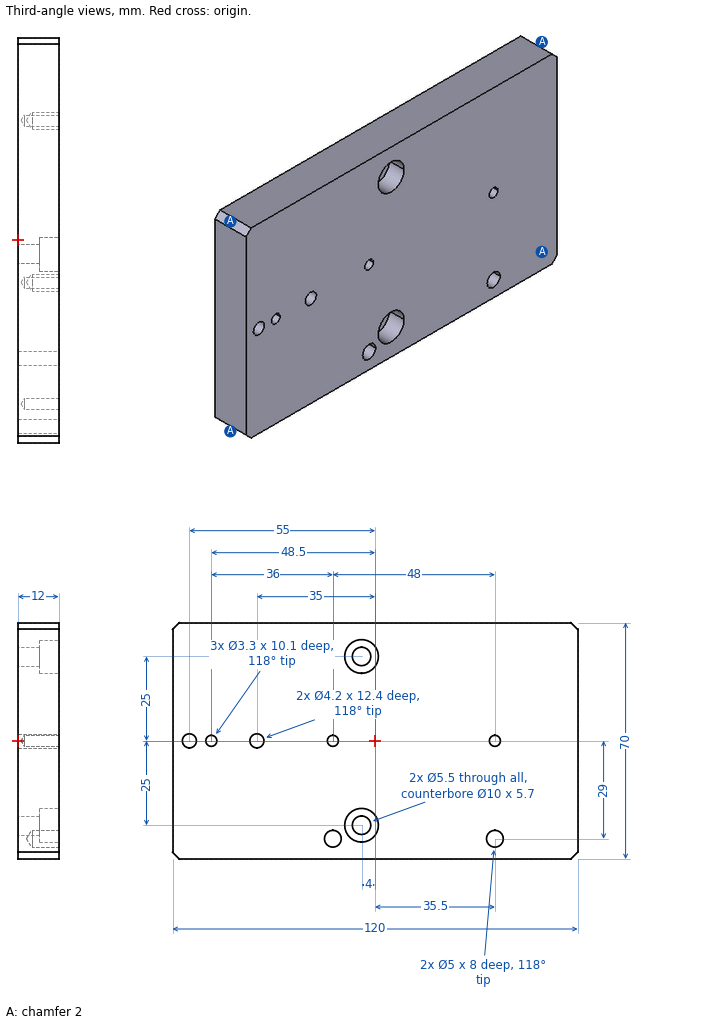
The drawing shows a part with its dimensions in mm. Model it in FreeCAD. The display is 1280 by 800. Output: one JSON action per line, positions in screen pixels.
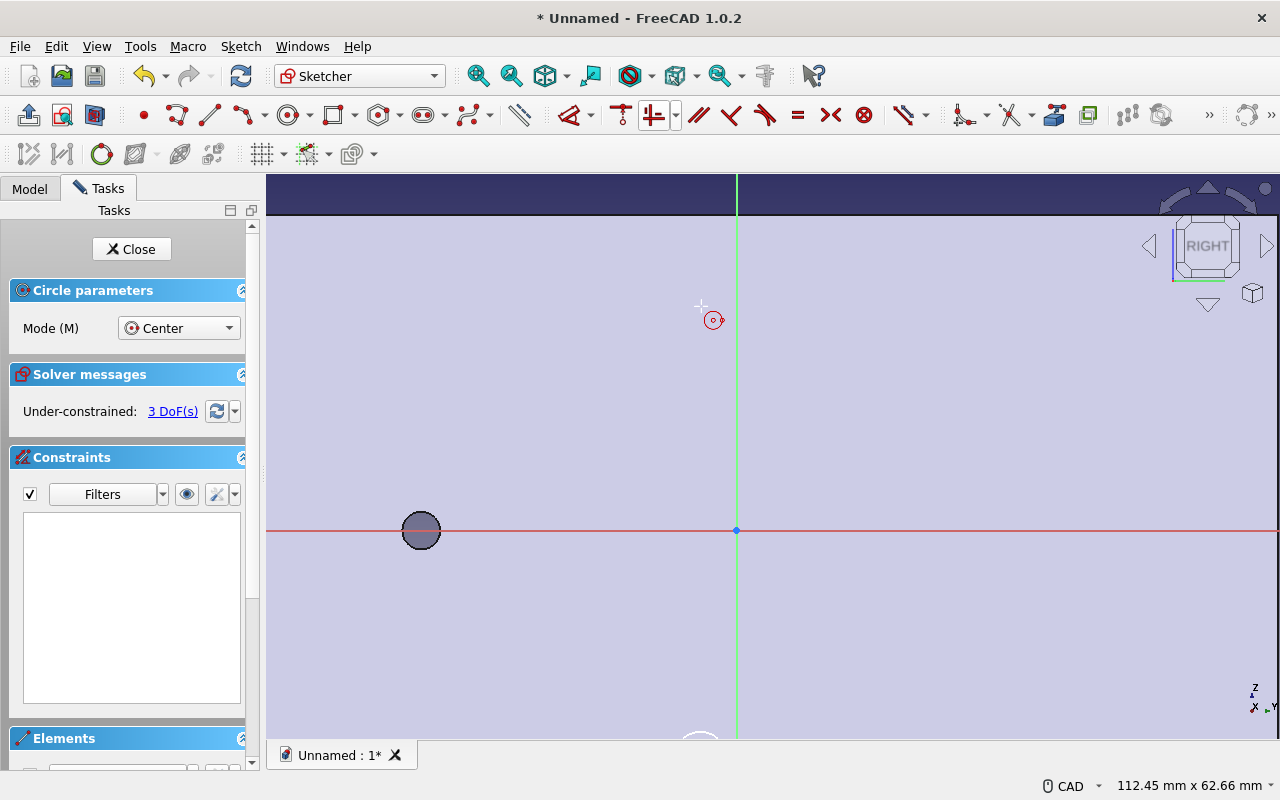
{"action": "left_click", "coordinate": [701, 305]}
{"action": "left_click", "coordinate": [718, 288]}
{"action": "key", "text": "Escape"}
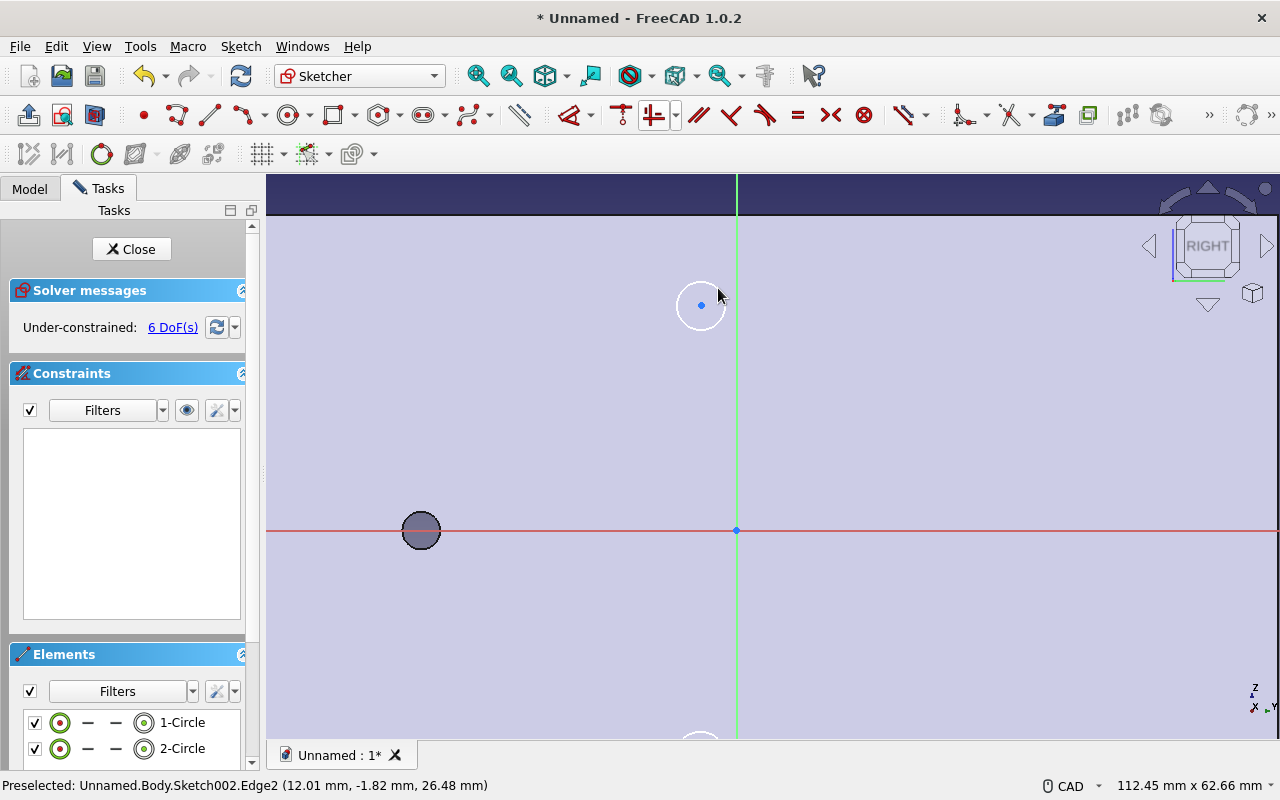
{"action": "scroll", "coordinate": [701, 306], "scroll_direction": "down", "scroll_amount": 2}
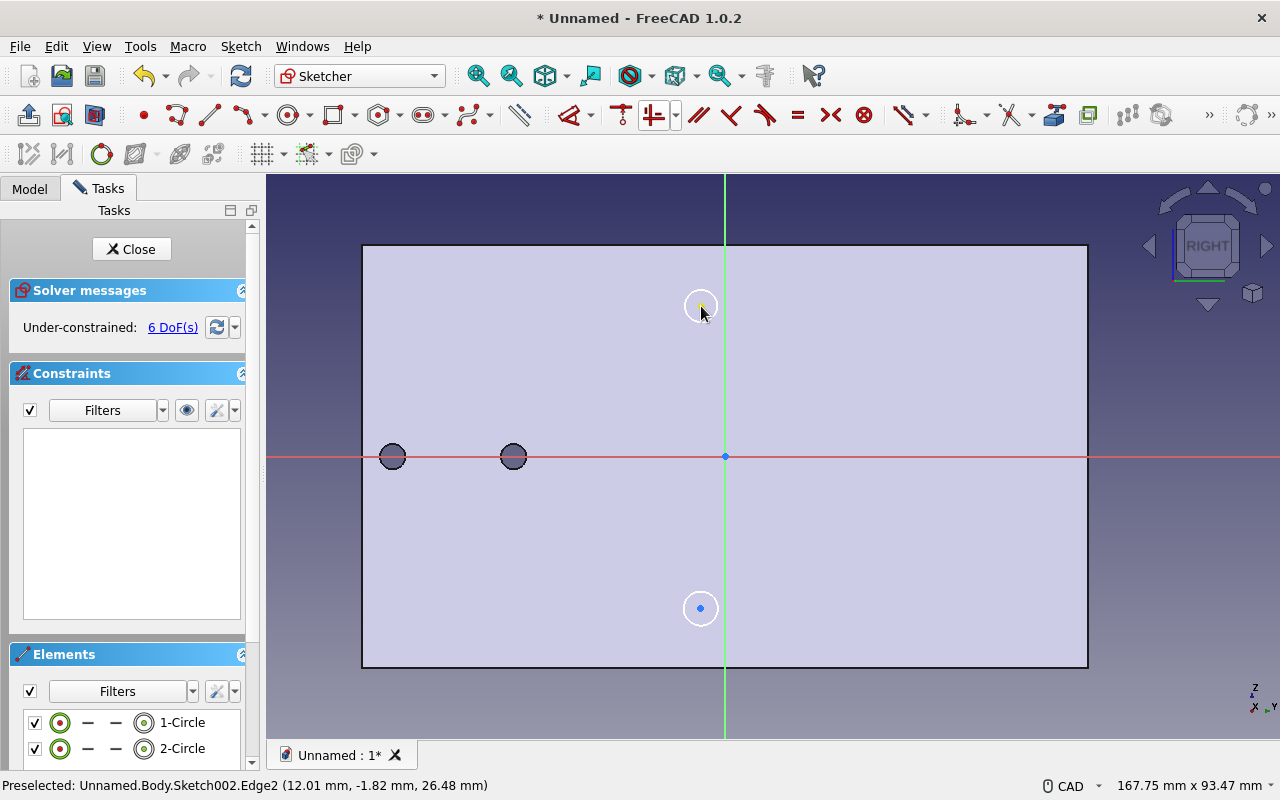
{"action": "left_click", "coordinate": [713, 596]}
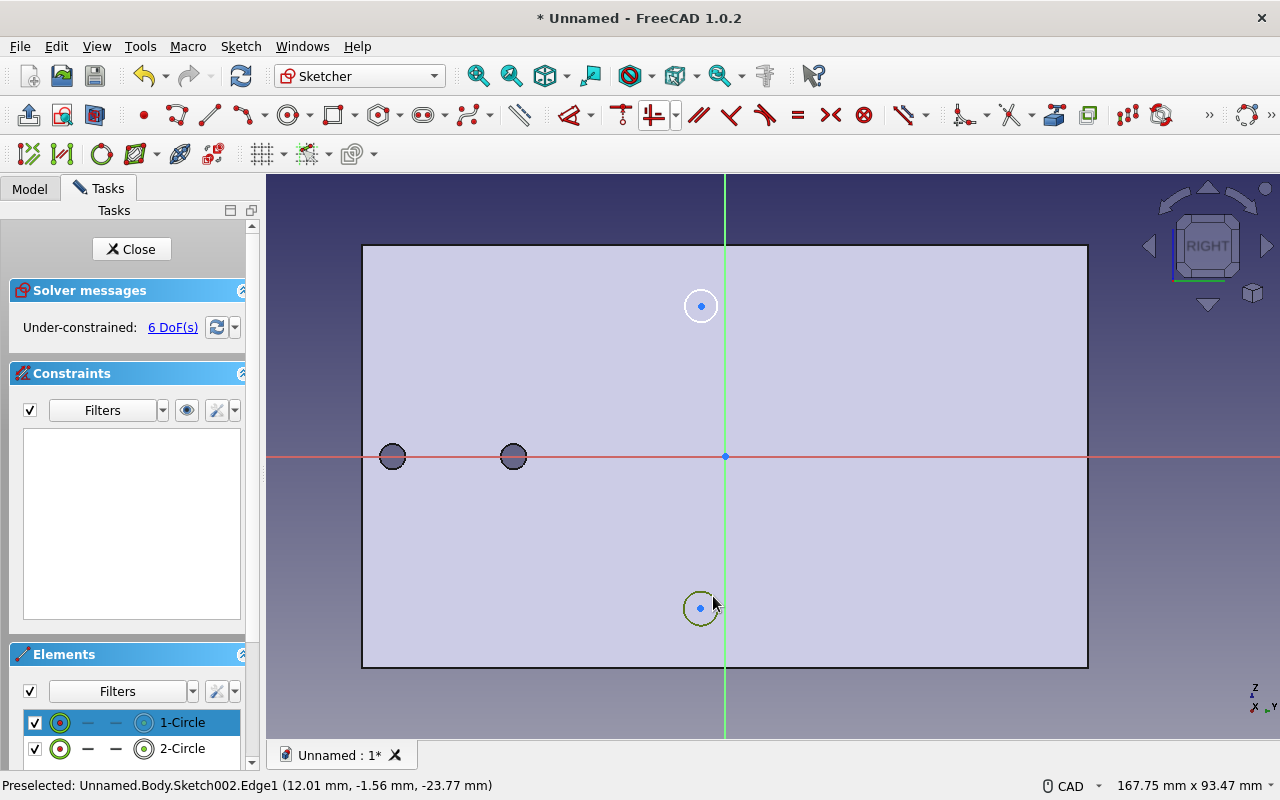
{"action": "left_click", "coordinate": [713, 295]}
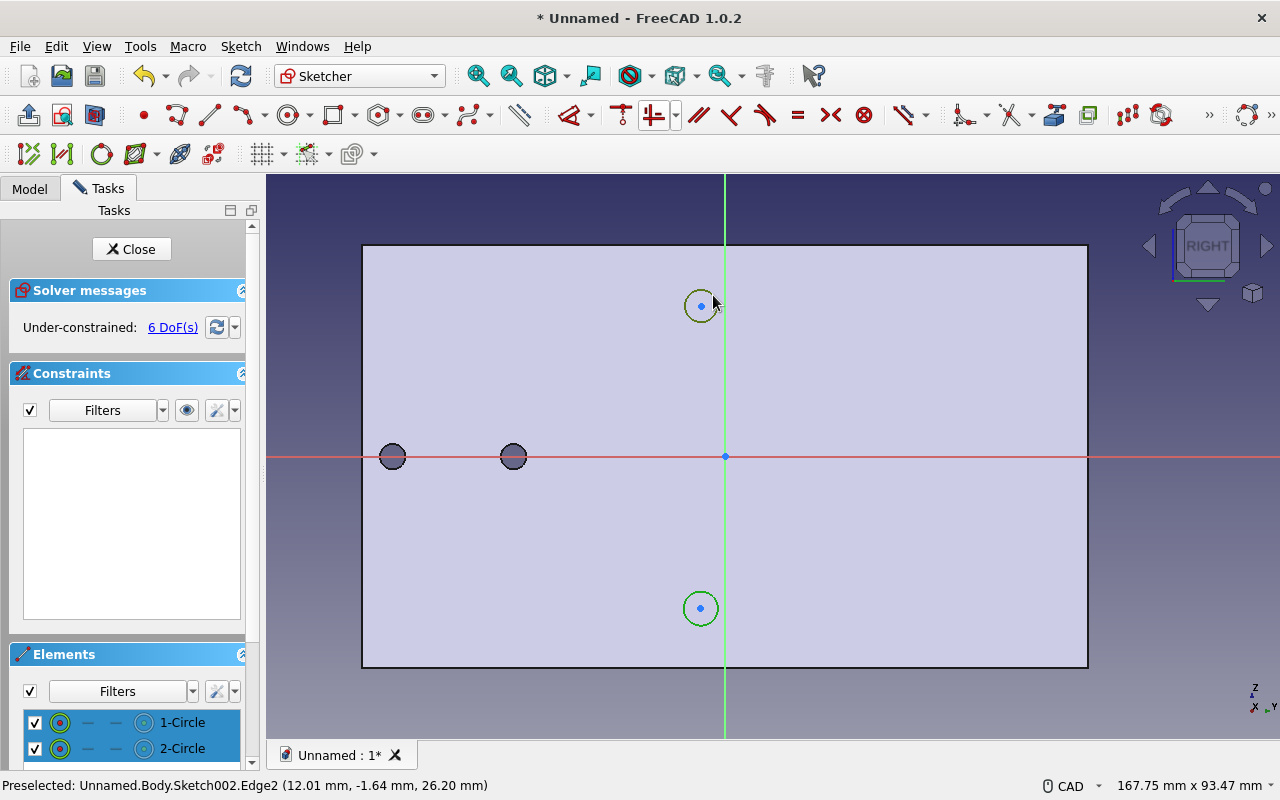
{"action": "left_click", "coordinate": [798, 116]}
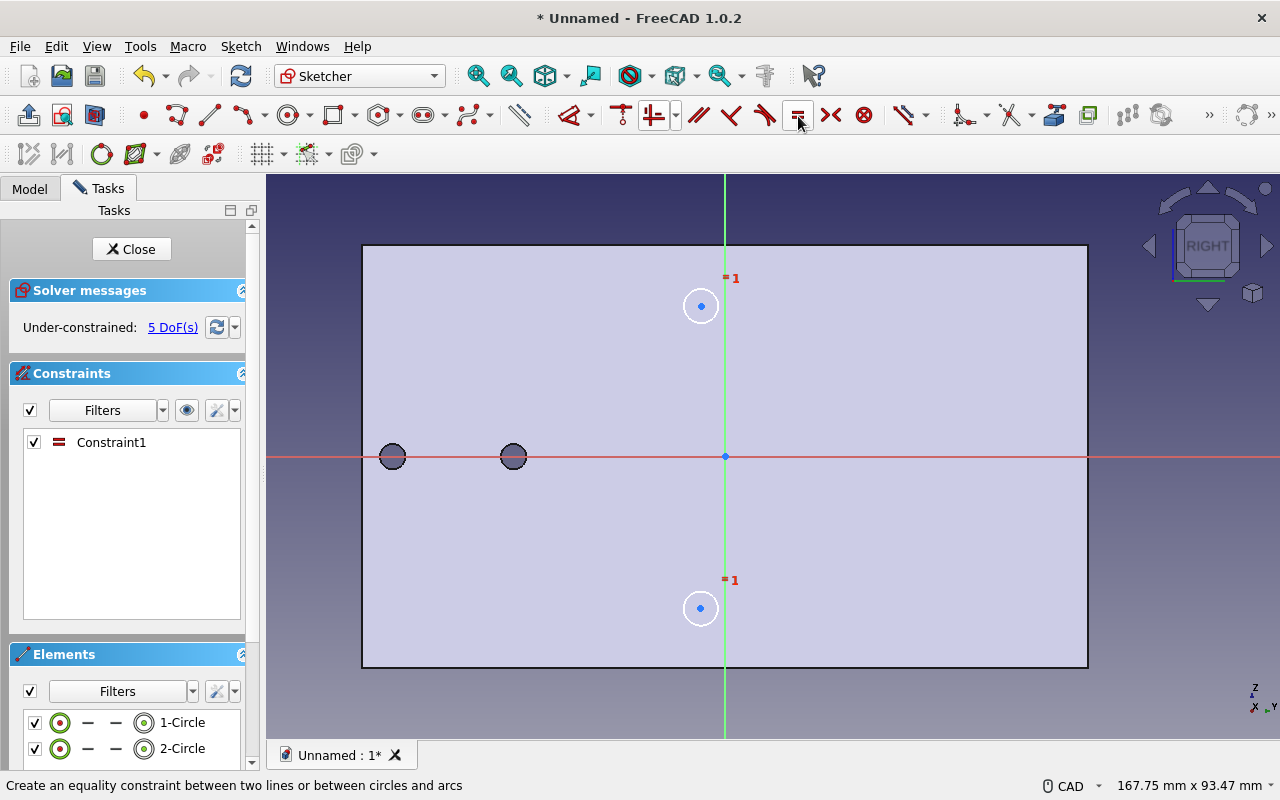
{"action": "left_click", "coordinate": [701, 609]}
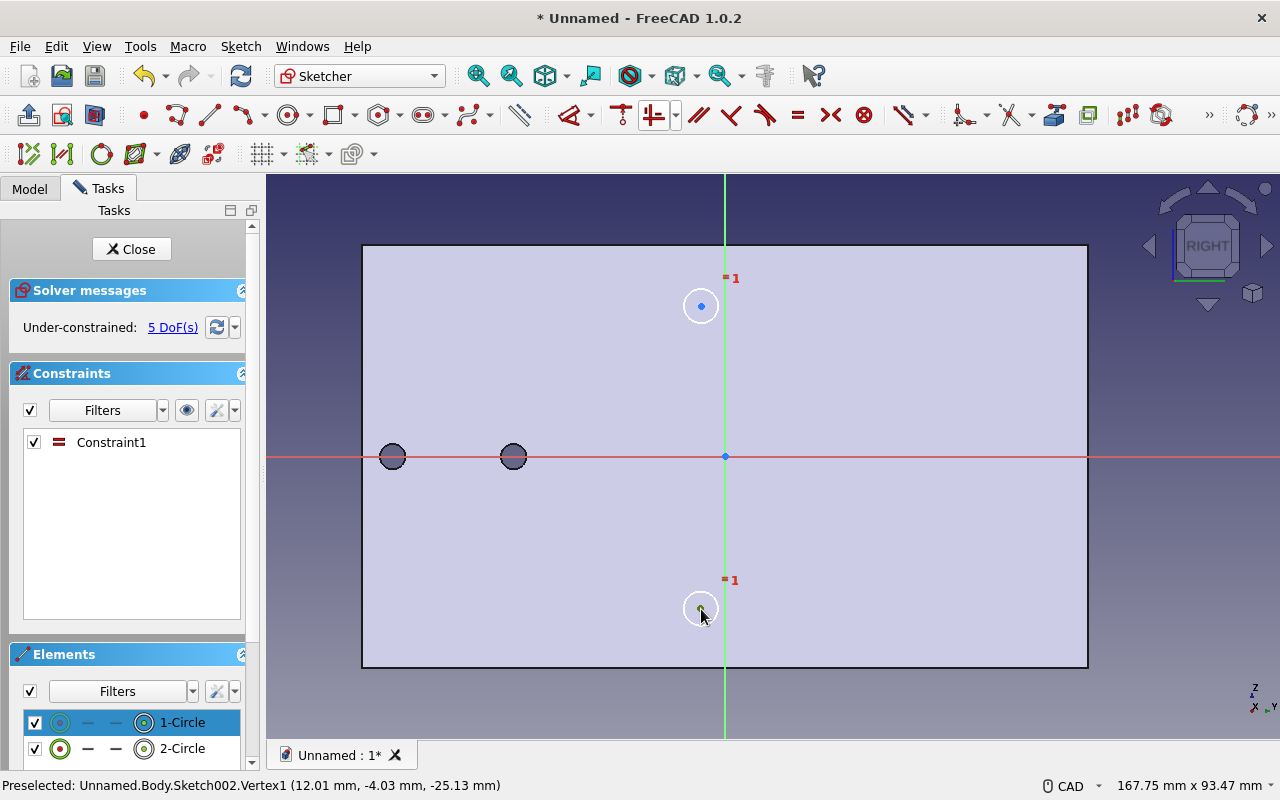
{"action": "left_click", "coordinate": [701, 306]}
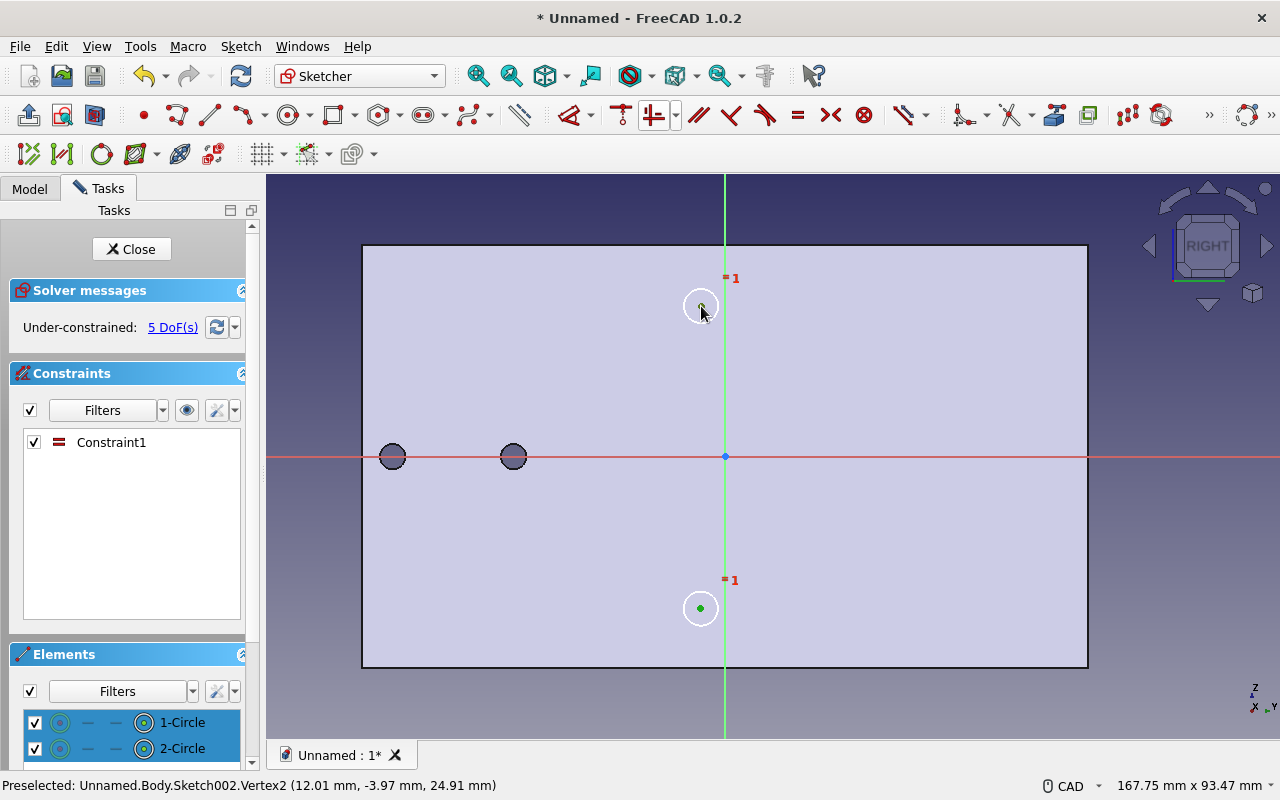
{"action": "key", "text": "v"}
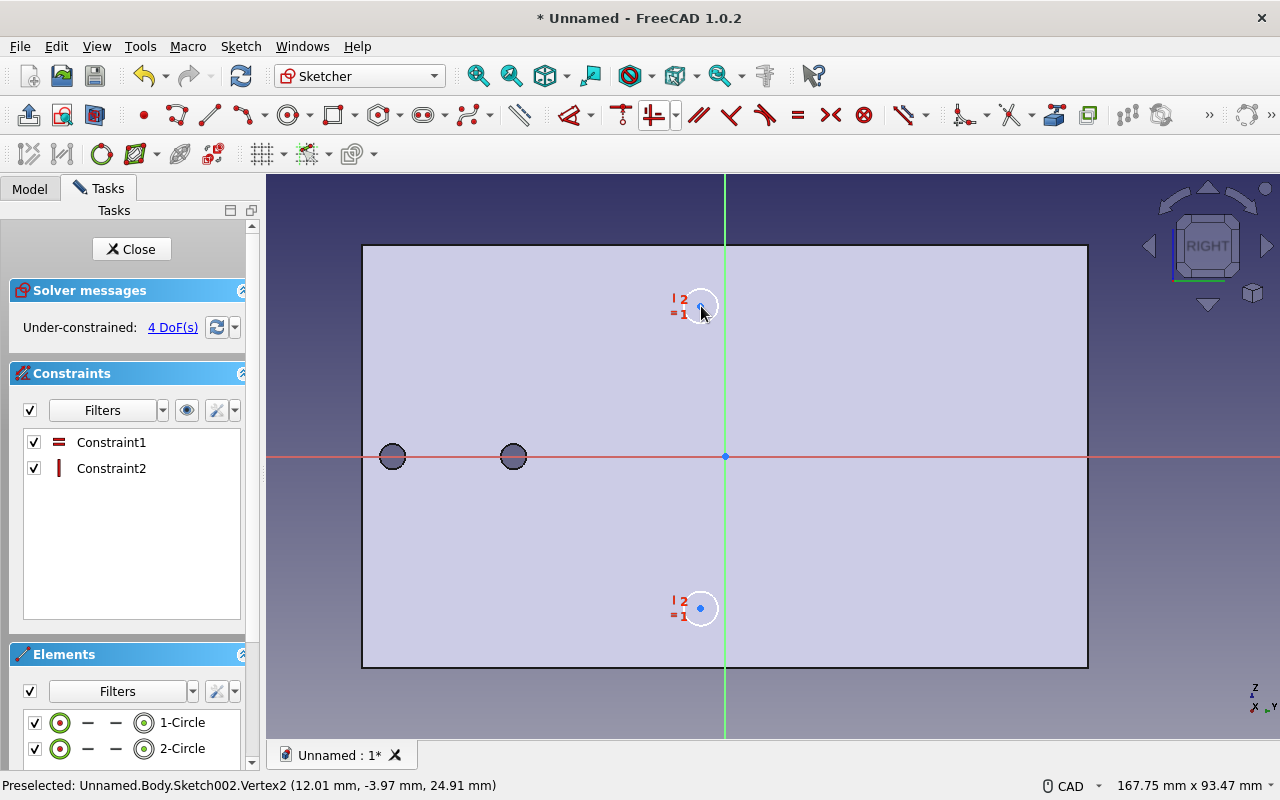
{"action": "left_click", "coordinate": [568, 116]}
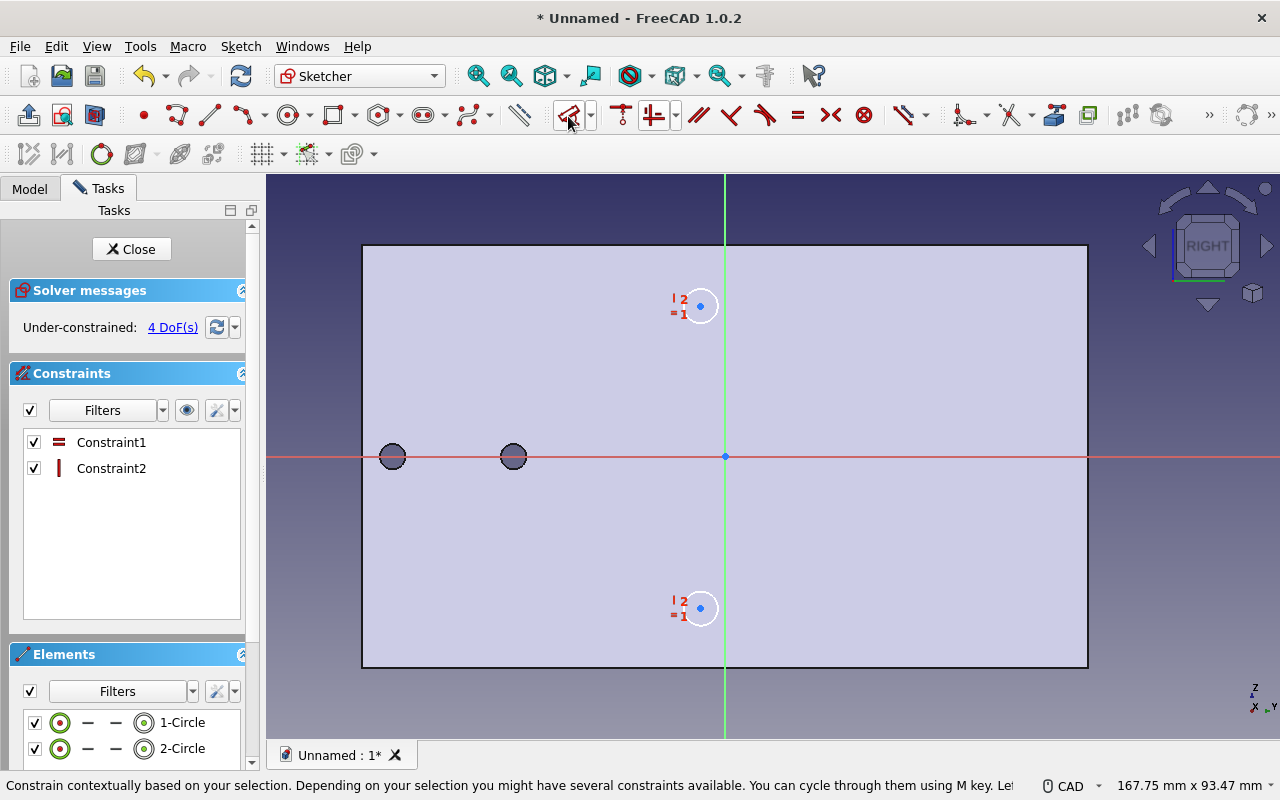
{"action": "left_click", "coordinate": [713, 596]}
{"action": "left_click", "coordinate": [748, 594]}